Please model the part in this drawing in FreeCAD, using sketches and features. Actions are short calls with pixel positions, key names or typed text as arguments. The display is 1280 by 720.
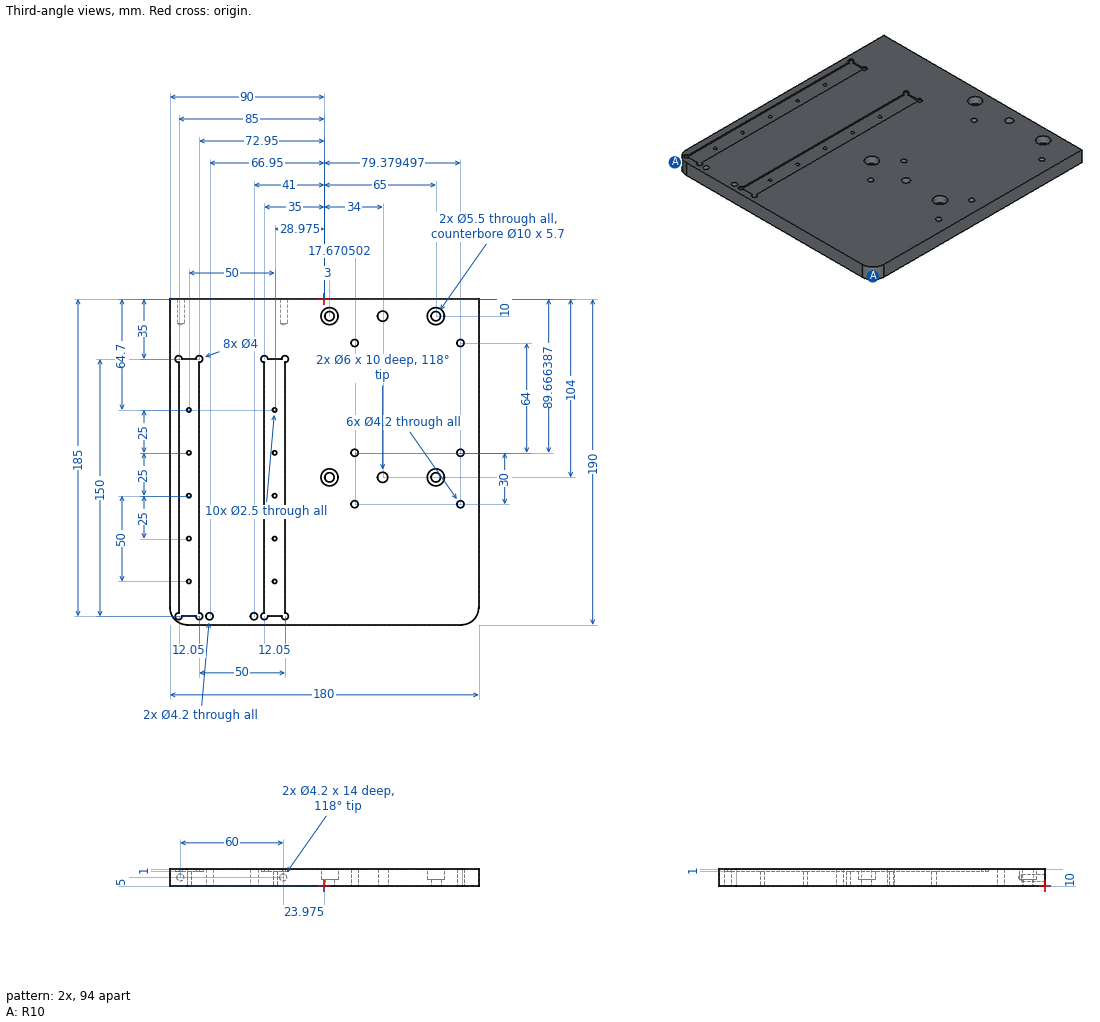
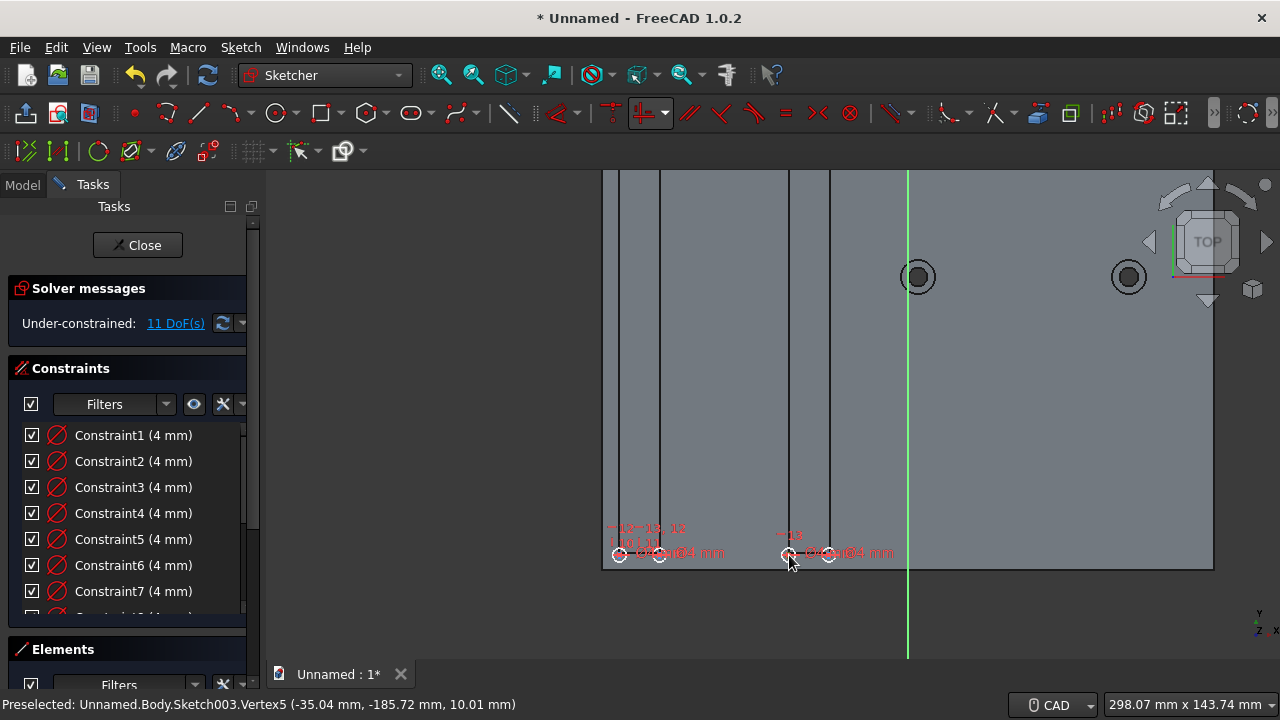
click(829, 555)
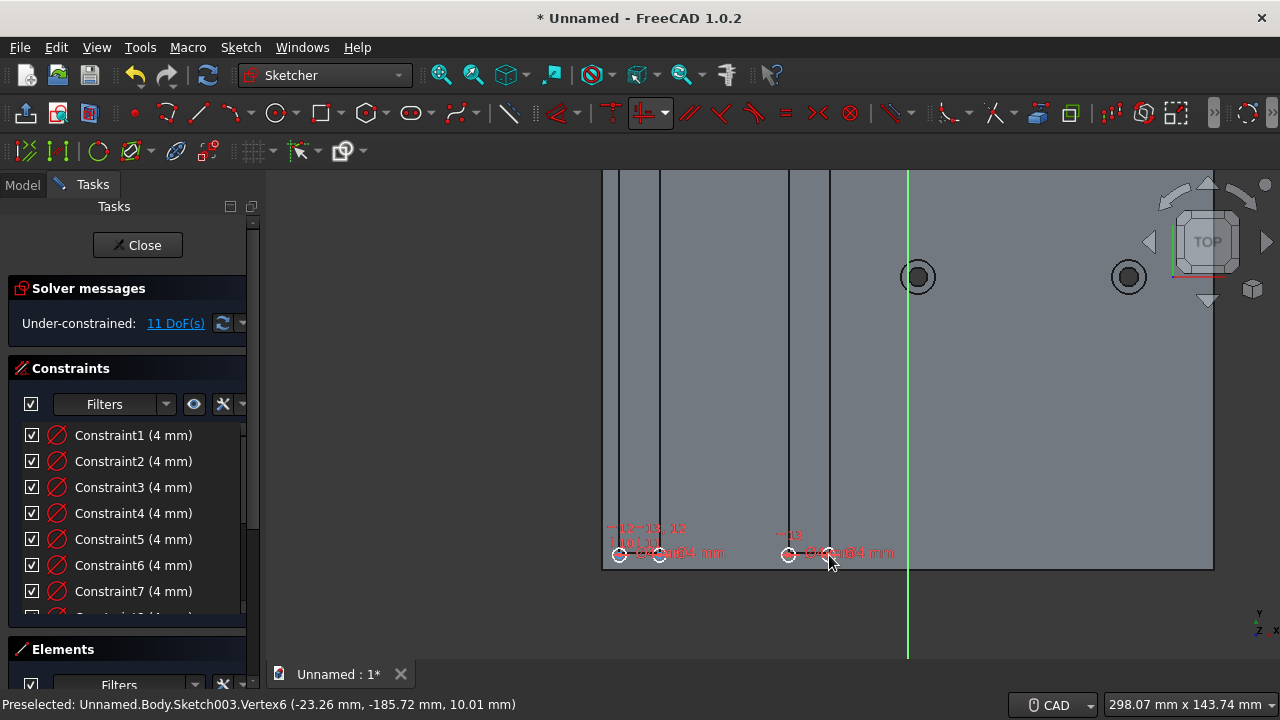
key(h)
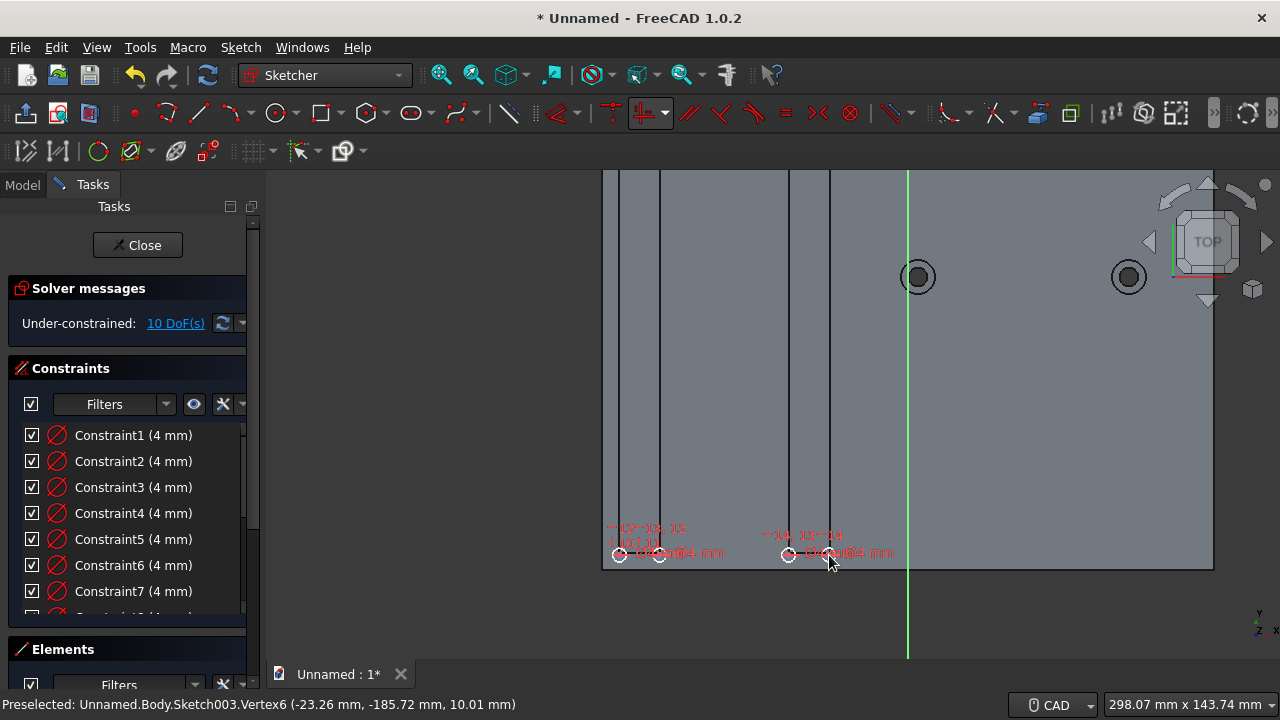
click(789, 555)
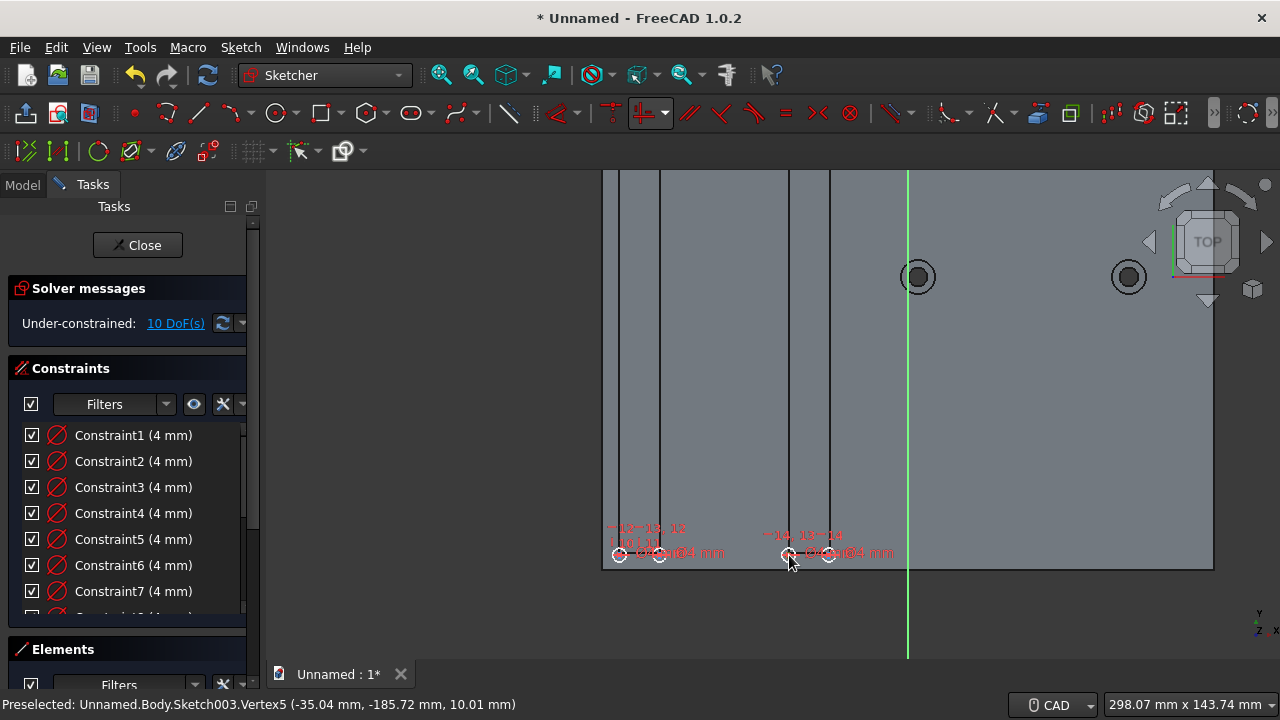
scroll(659, 556, down, 4)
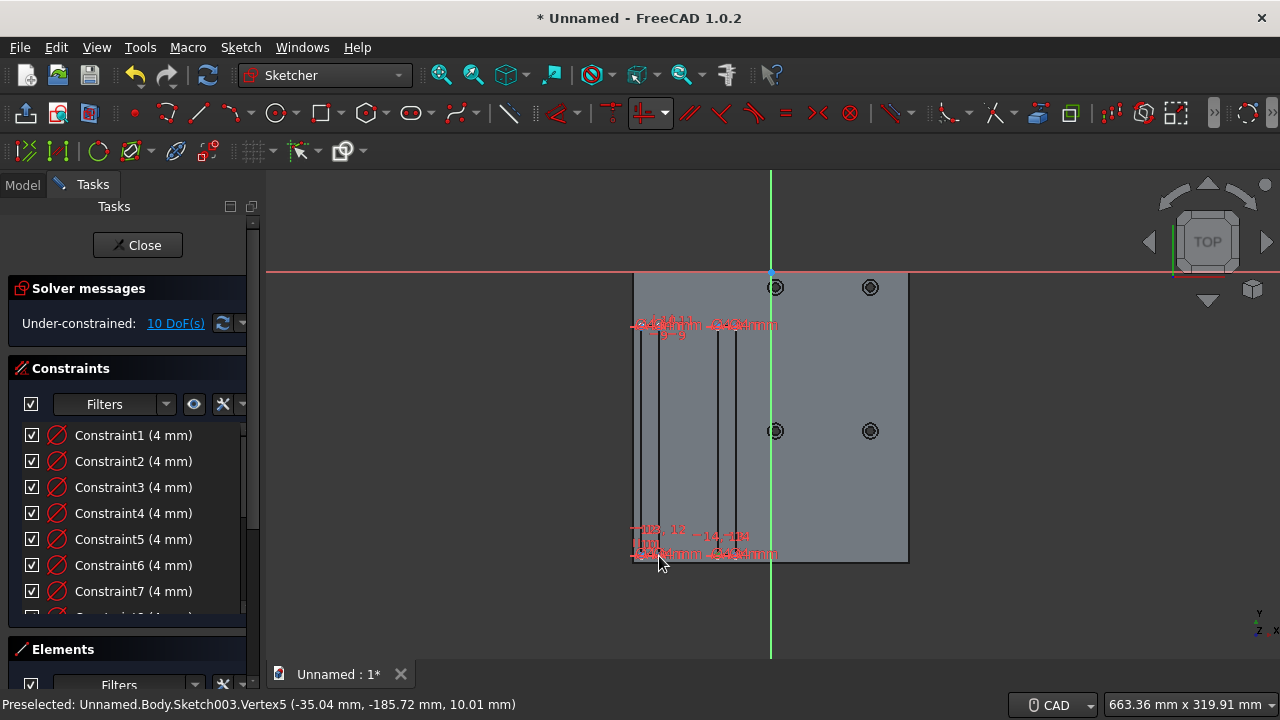
click(717, 327)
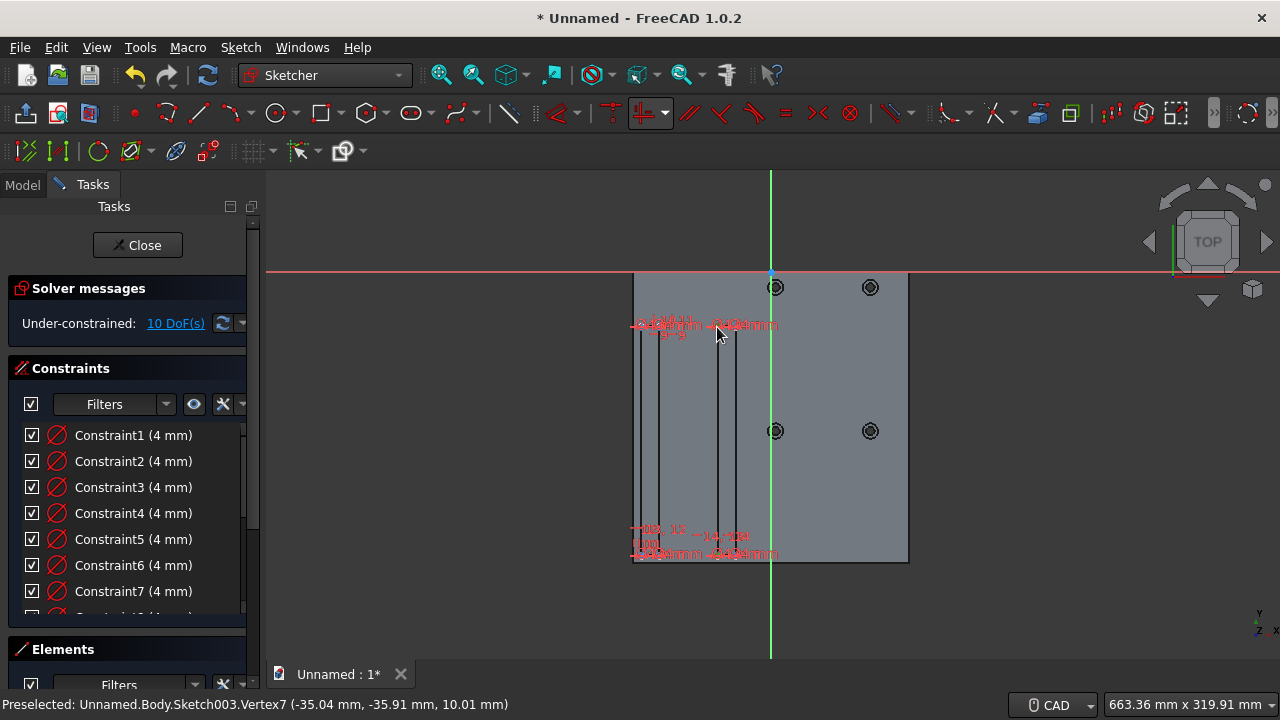
key(v)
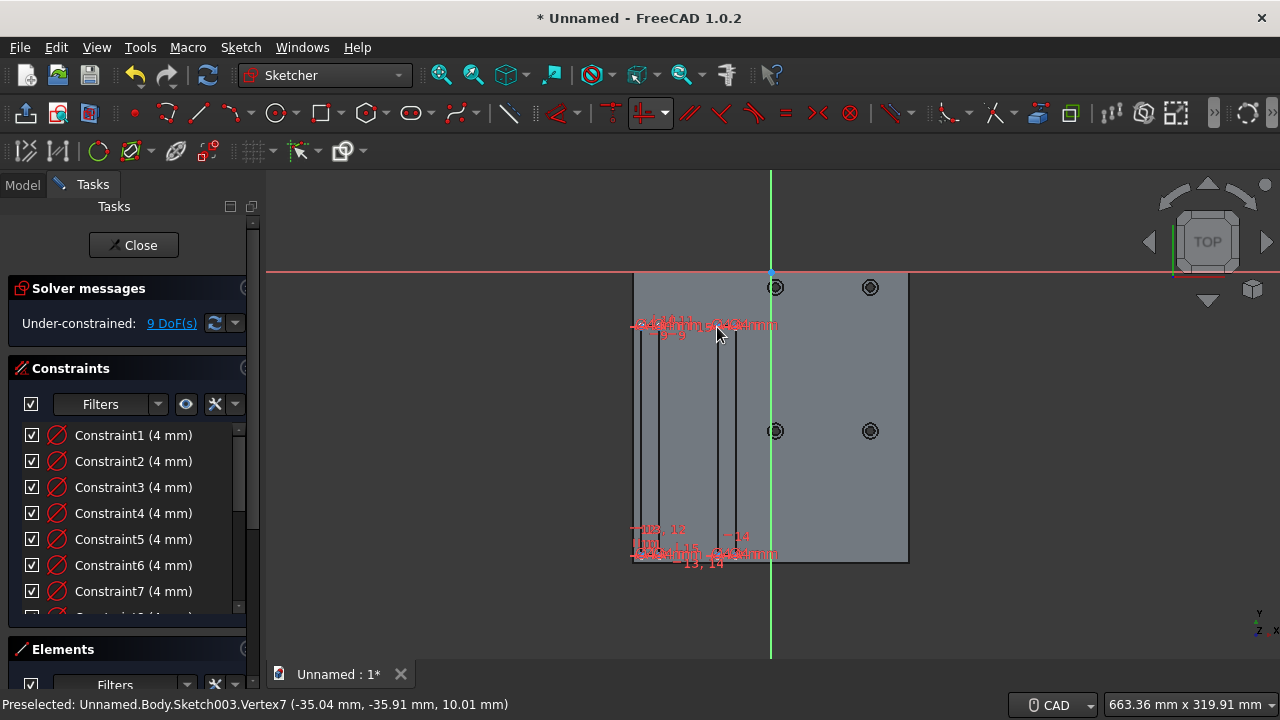
click(659, 327)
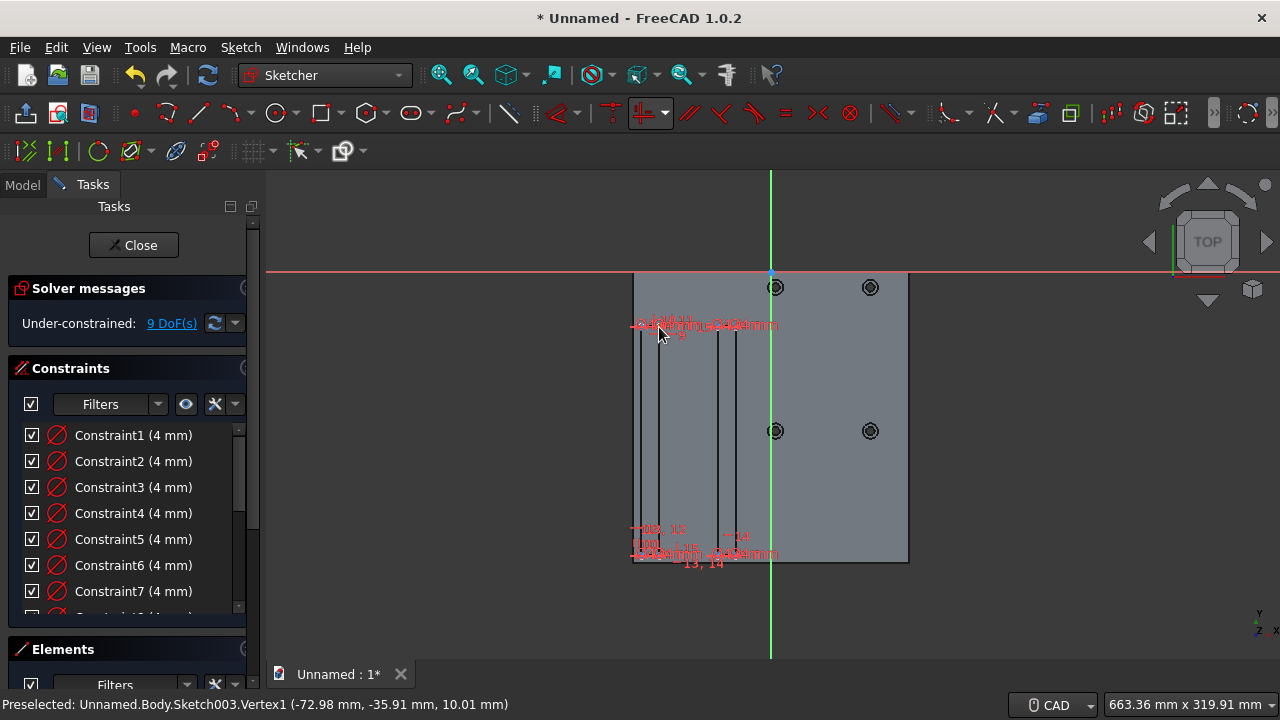
click(717, 327)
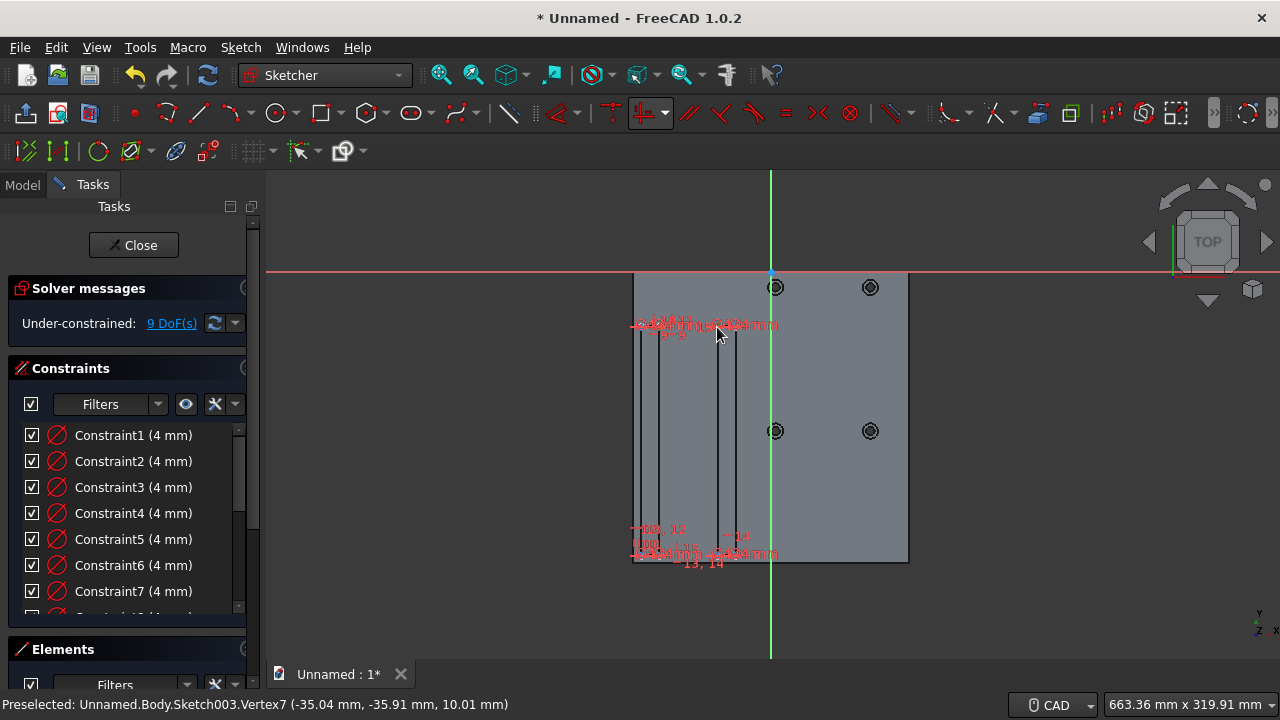
key(h)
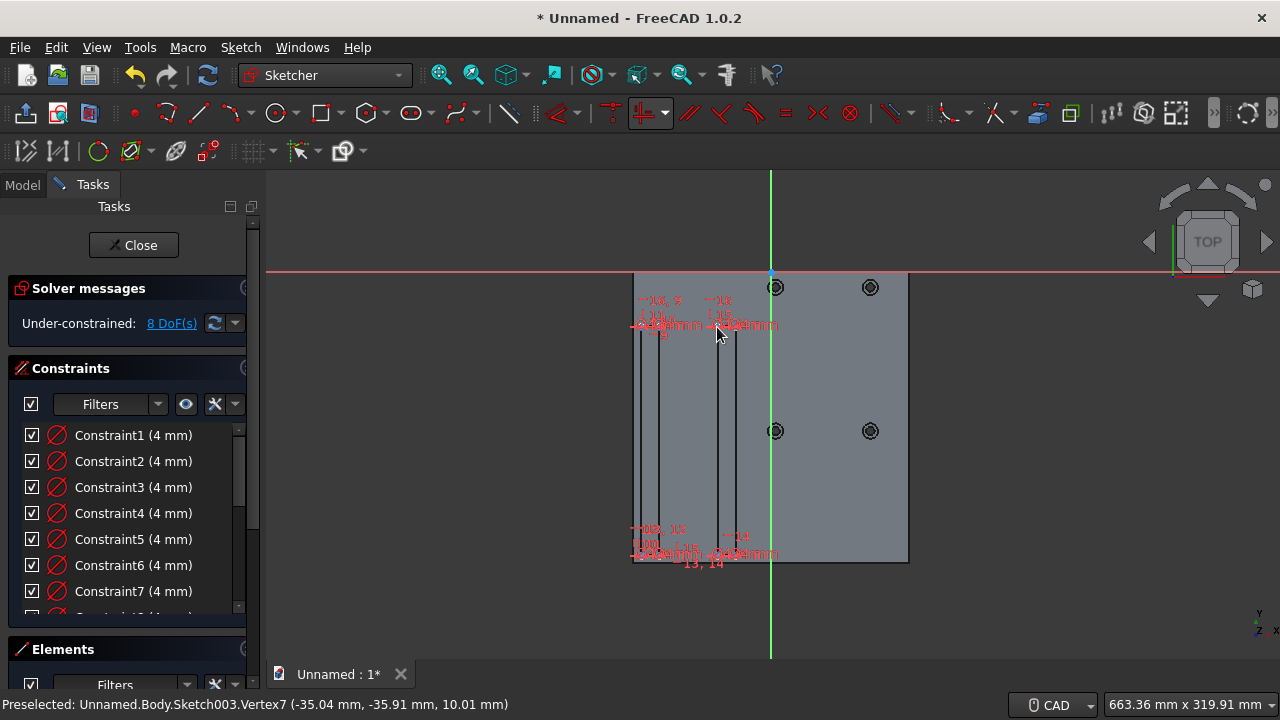
click(735, 556)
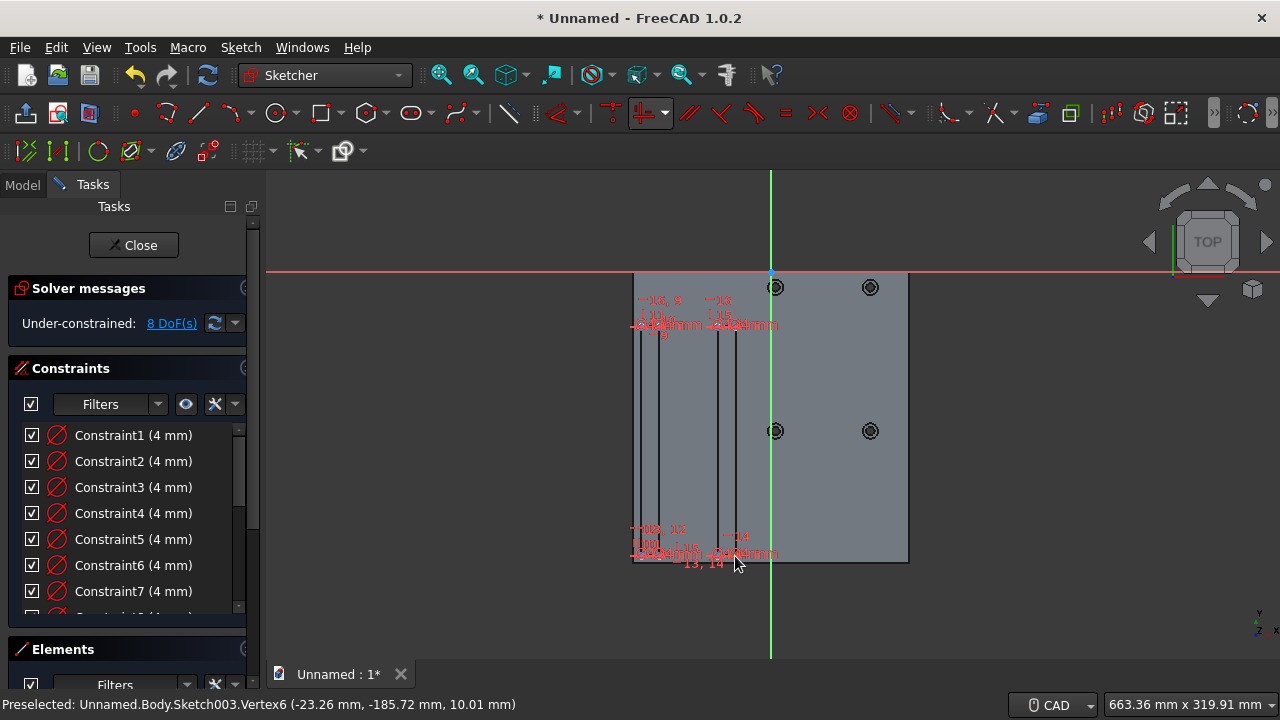
click(735, 327)